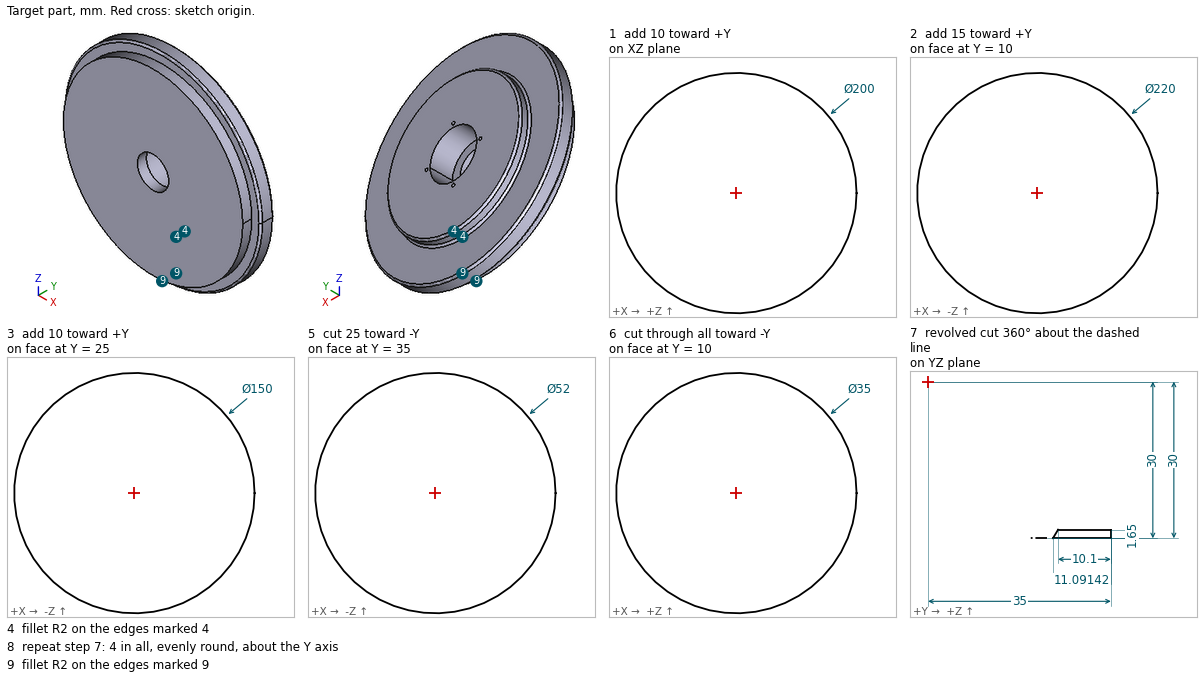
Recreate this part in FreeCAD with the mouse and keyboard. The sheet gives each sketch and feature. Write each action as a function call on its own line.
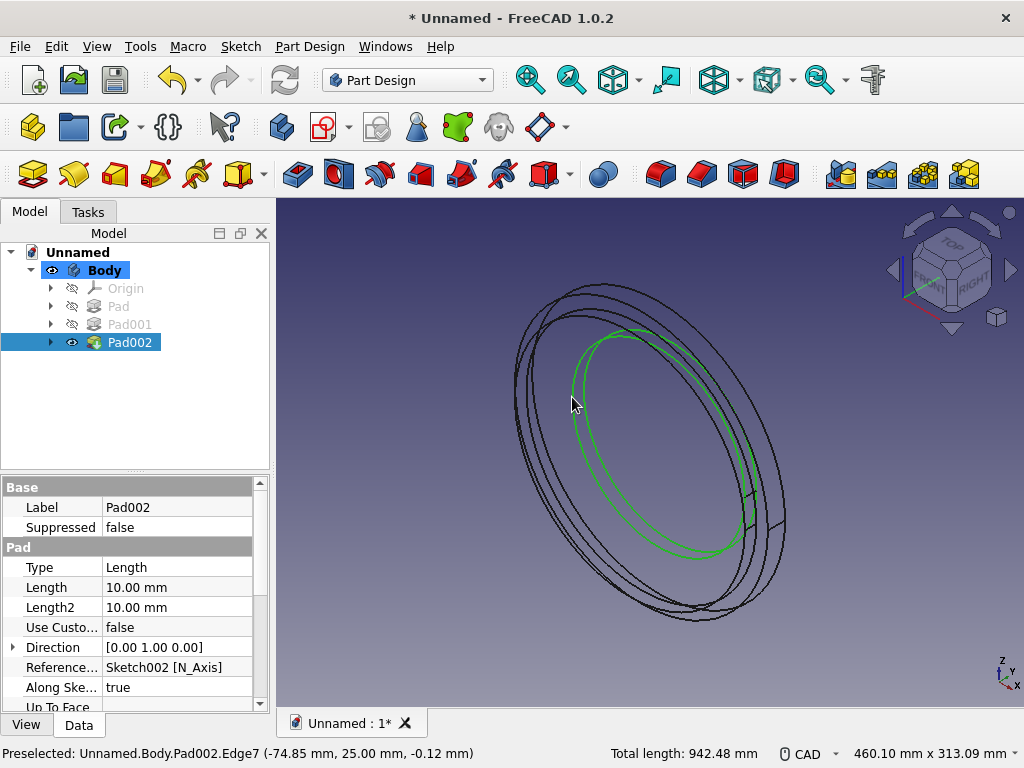
key(v)
key(1)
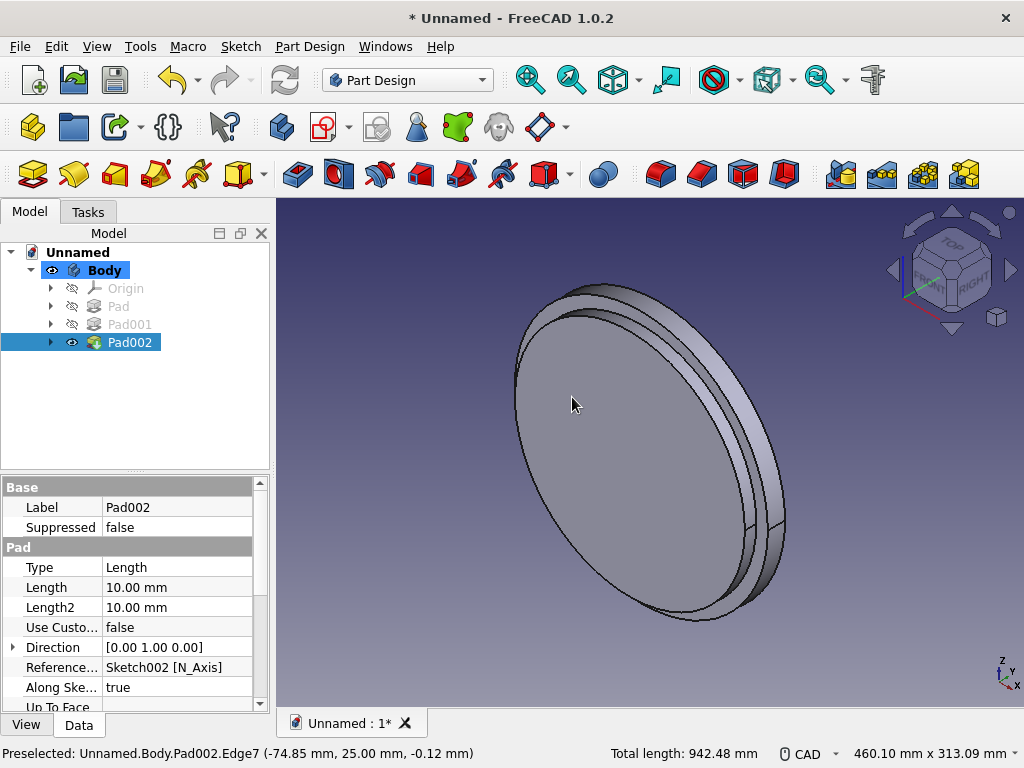
click(661, 174)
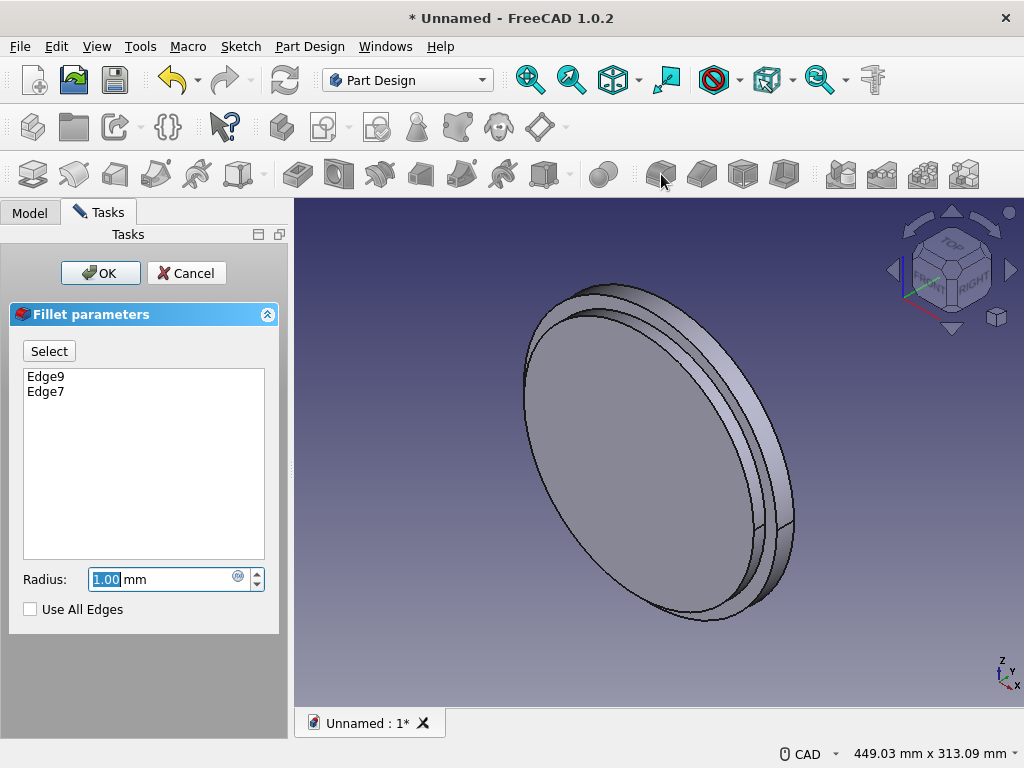
text(2)
key(Tab)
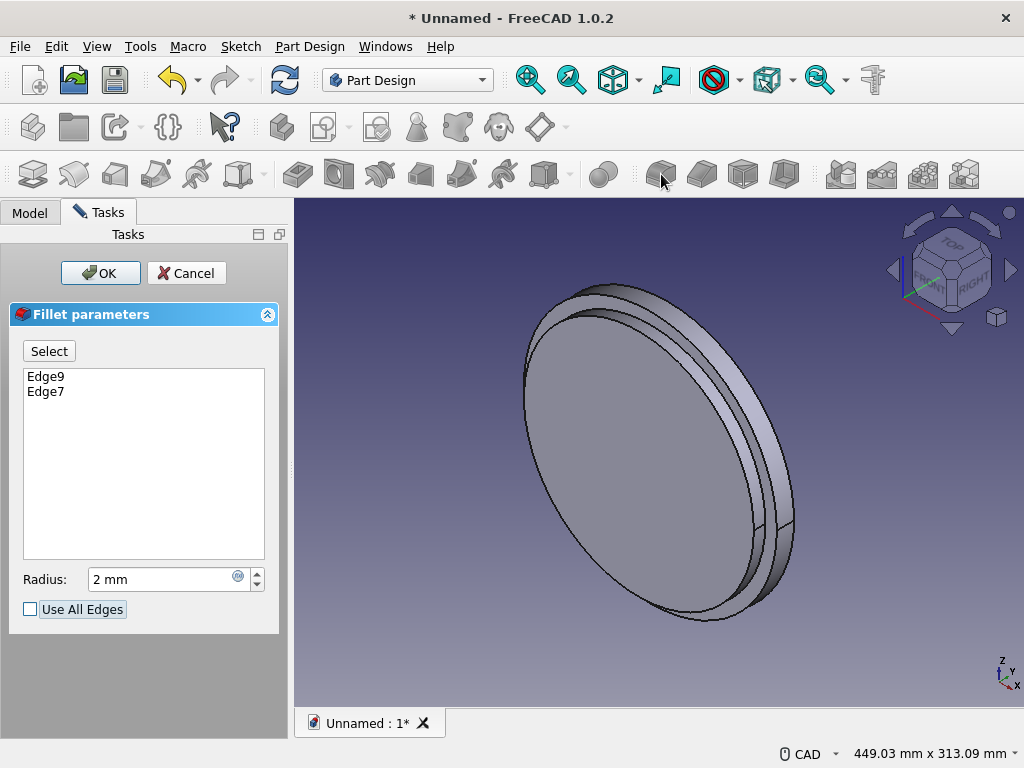
click(101, 273)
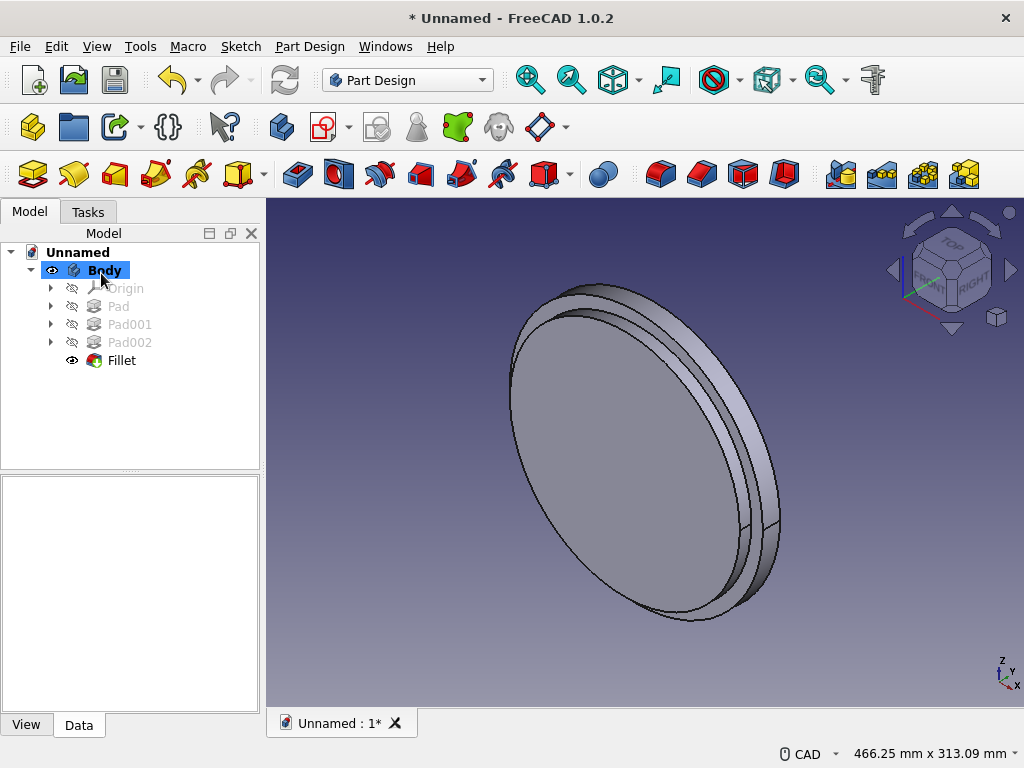
key(4)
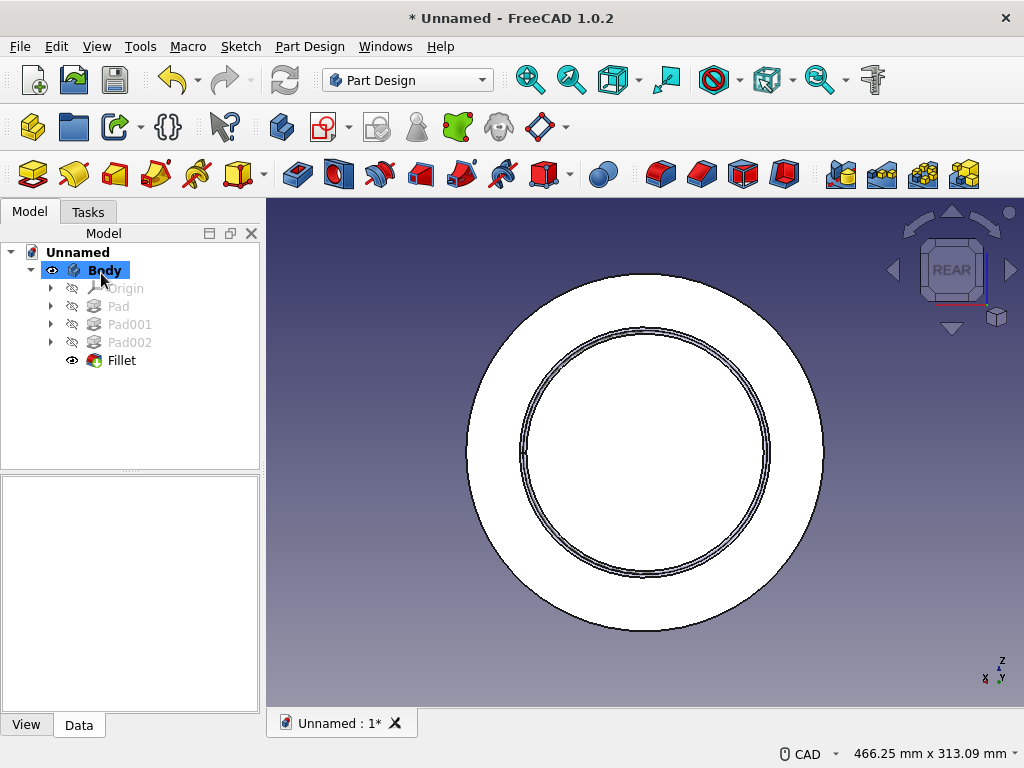
click(645, 451)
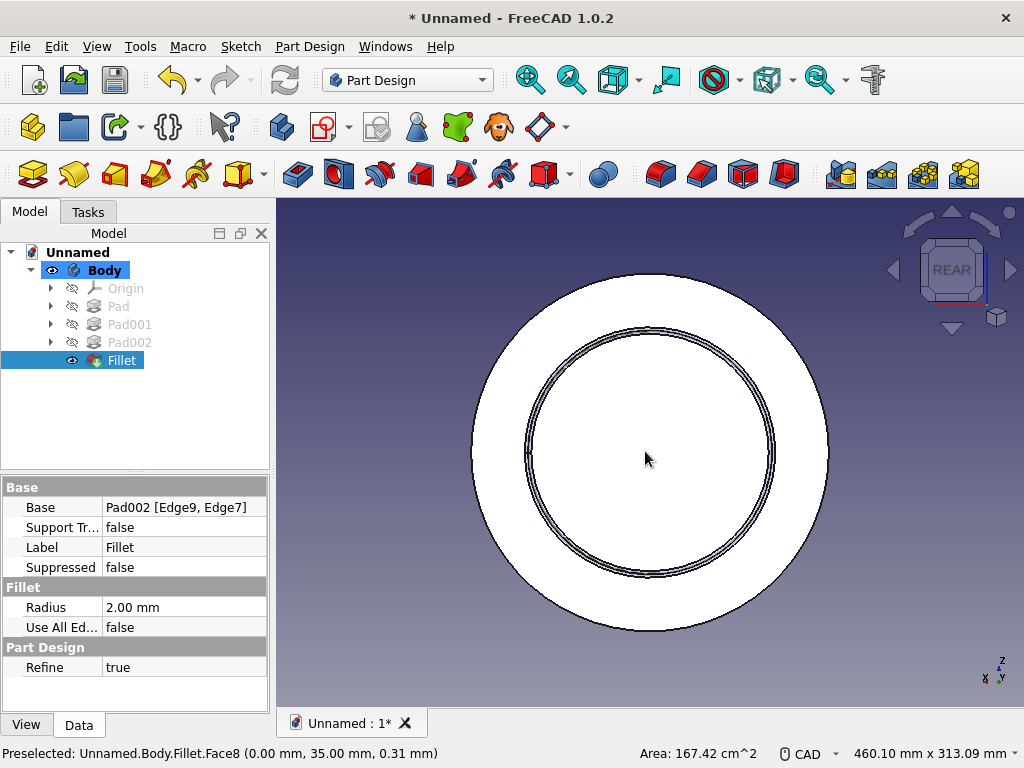
click(322, 128)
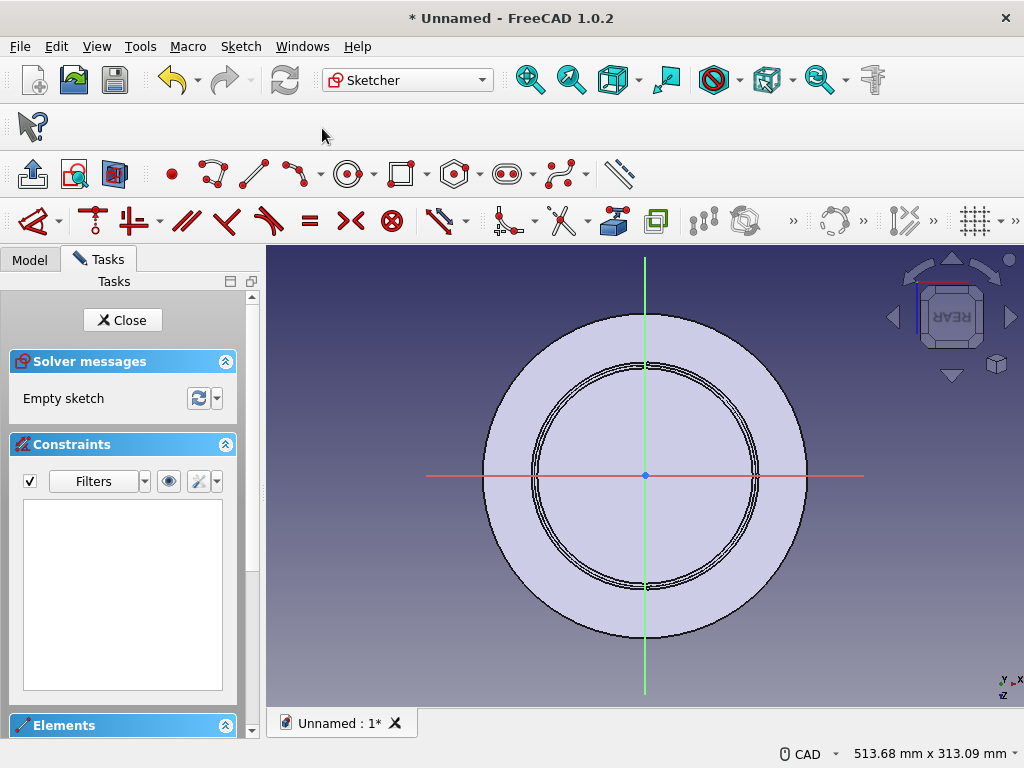
scroll(667, 476, up, 7)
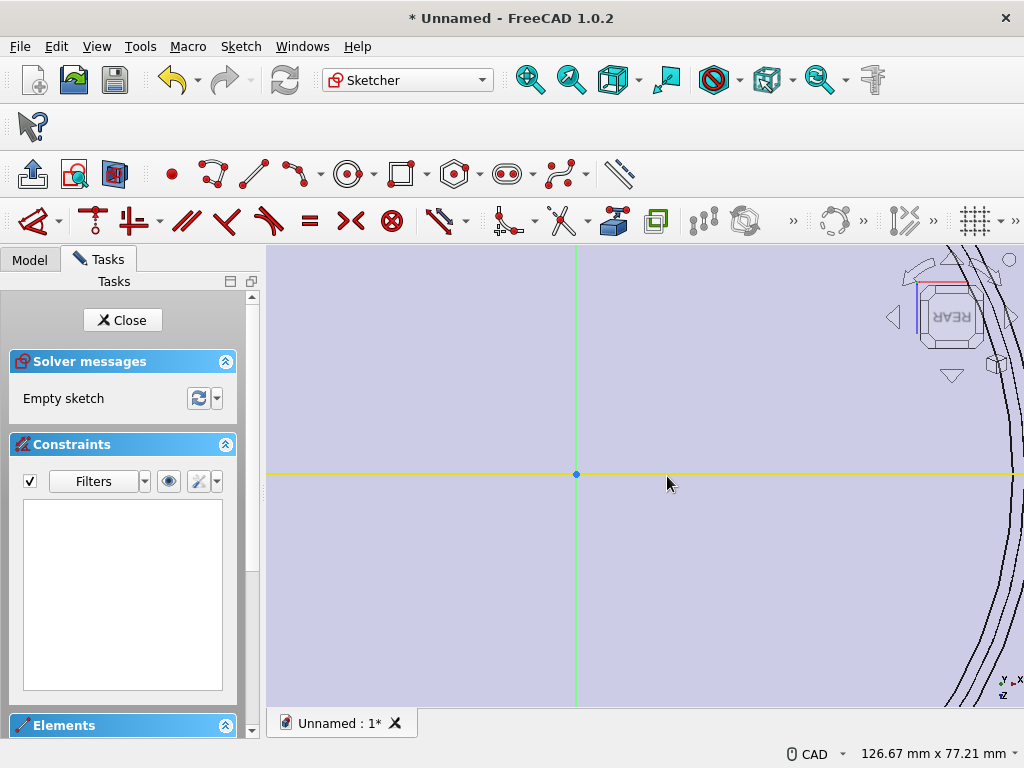
click(348, 174)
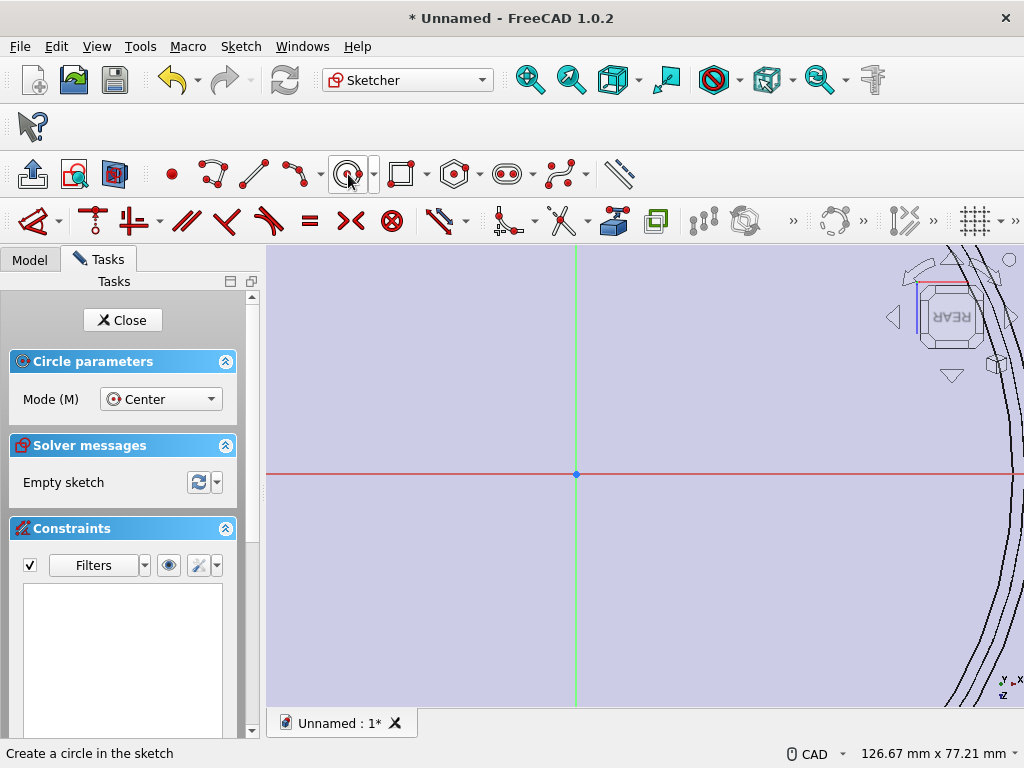
click(576, 474)
click(686, 364)
key(Escape)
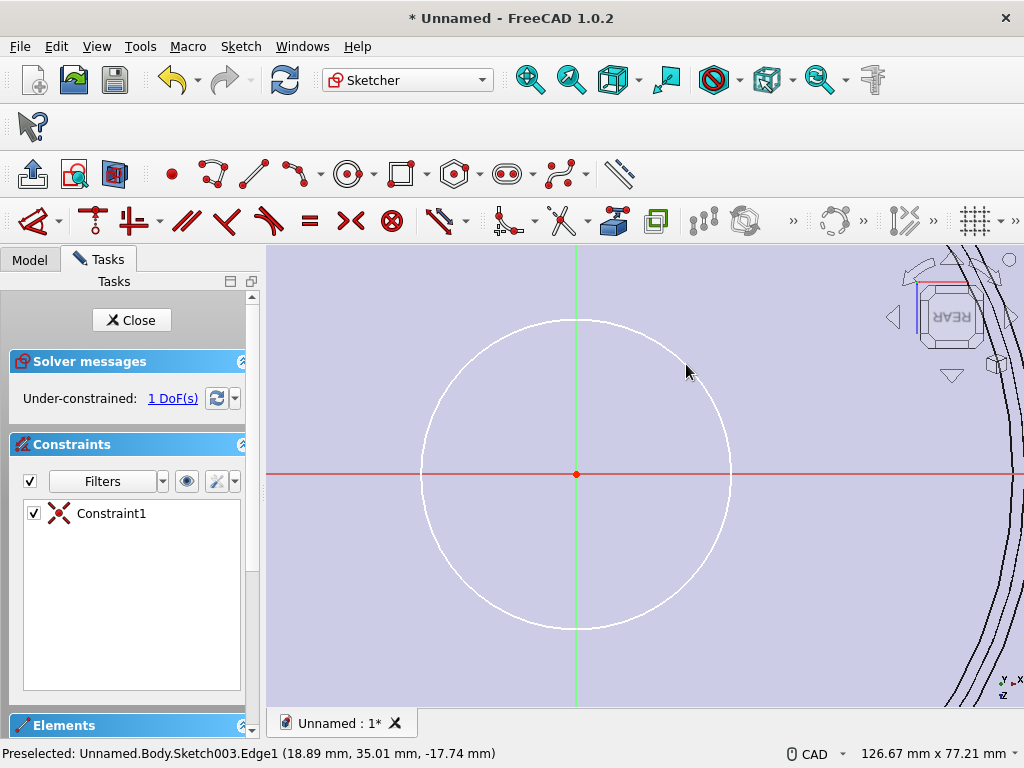
click(32, 222)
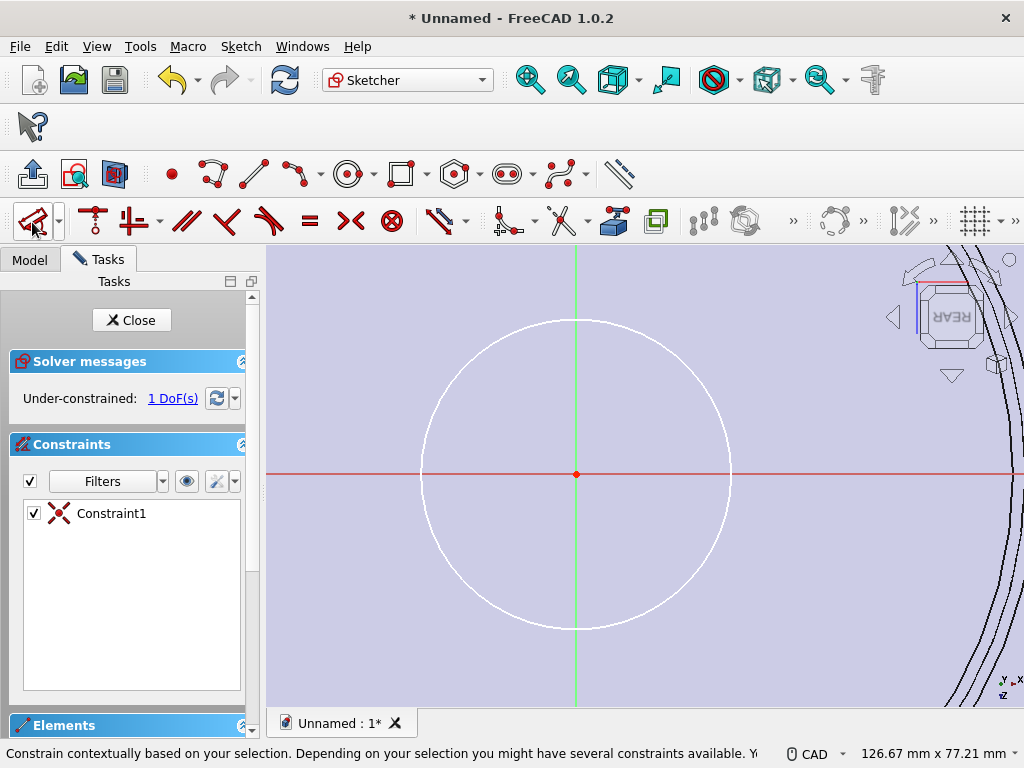
click(685, 364)
click(707, 341)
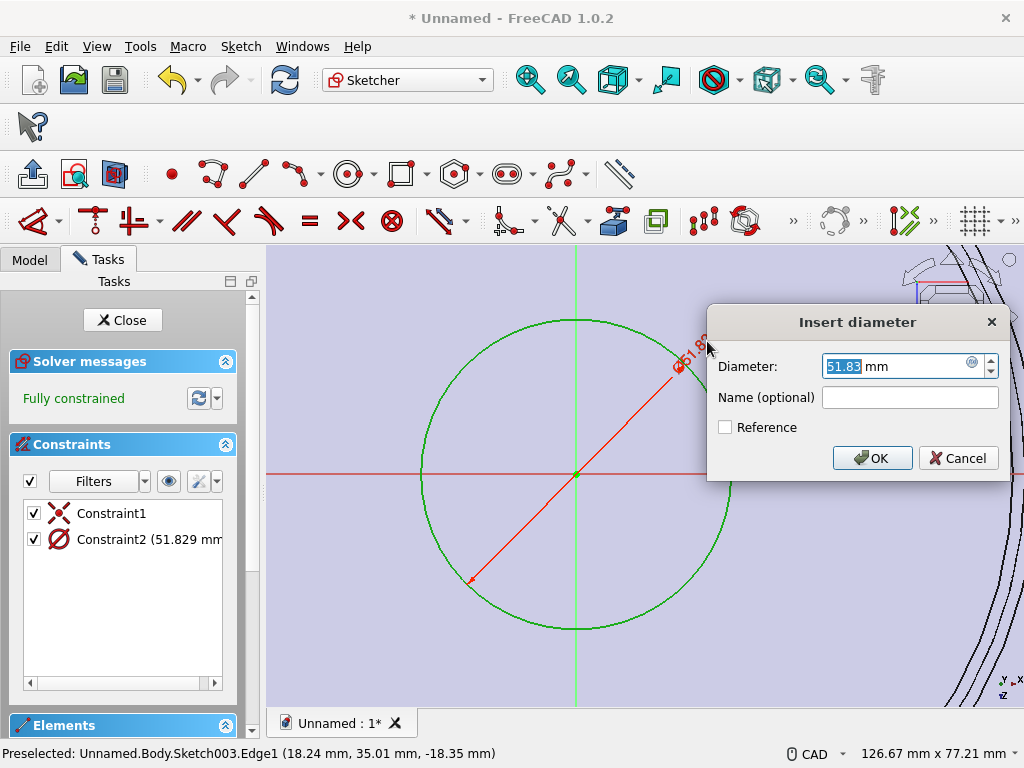
text(52)
key(Return)
key(Escape)